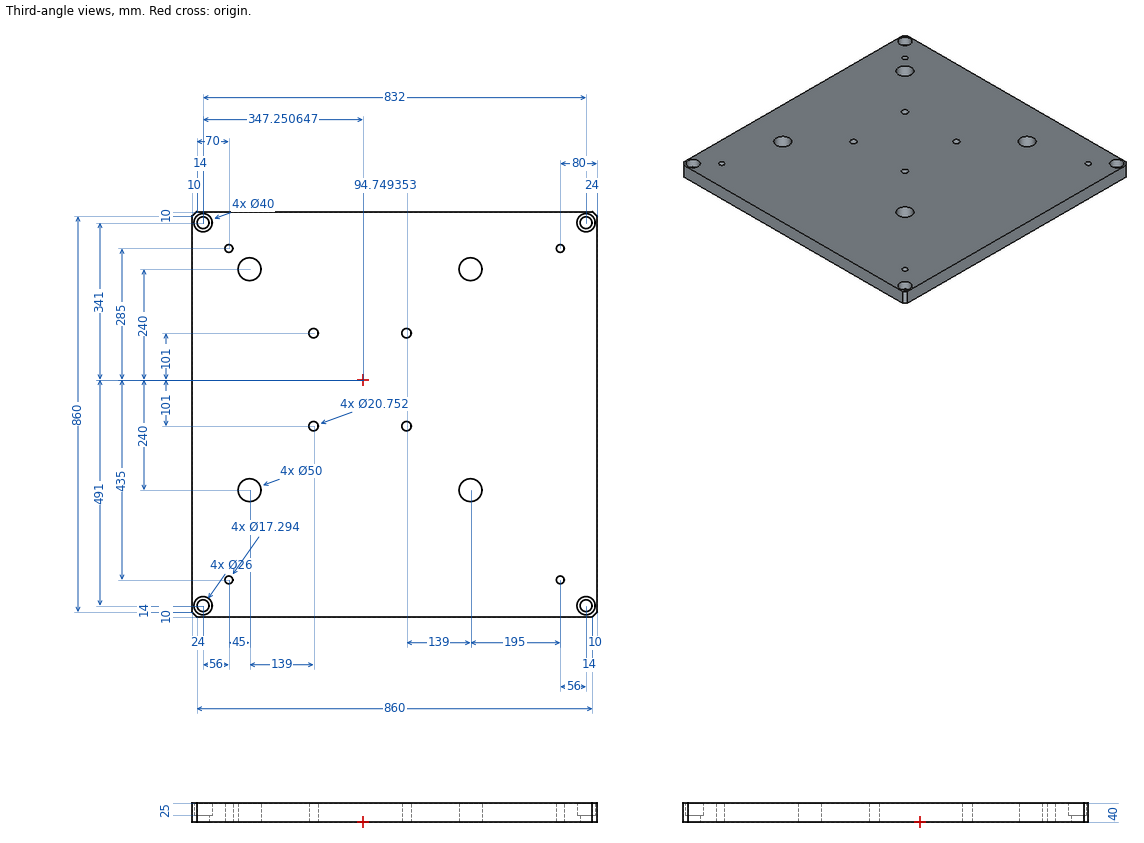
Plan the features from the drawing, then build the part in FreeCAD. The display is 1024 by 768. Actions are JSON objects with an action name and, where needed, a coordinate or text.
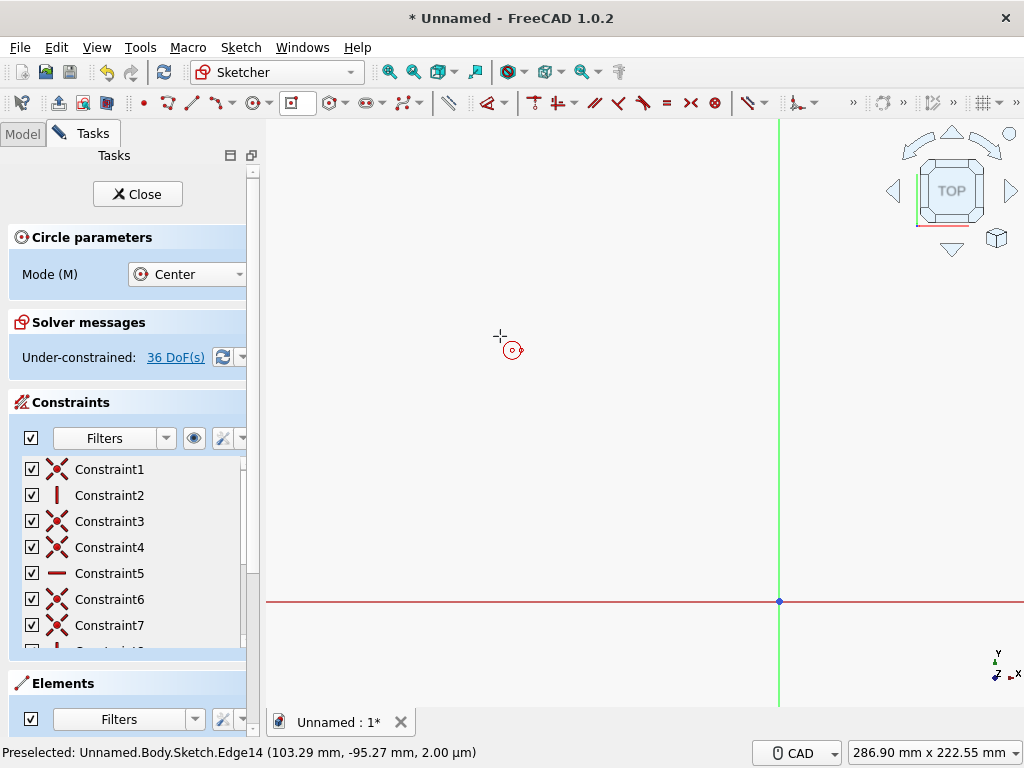
{"action": "scroll", "coordinate": [500, 336], "scroll_direction": "down", "scroll_amount": 9}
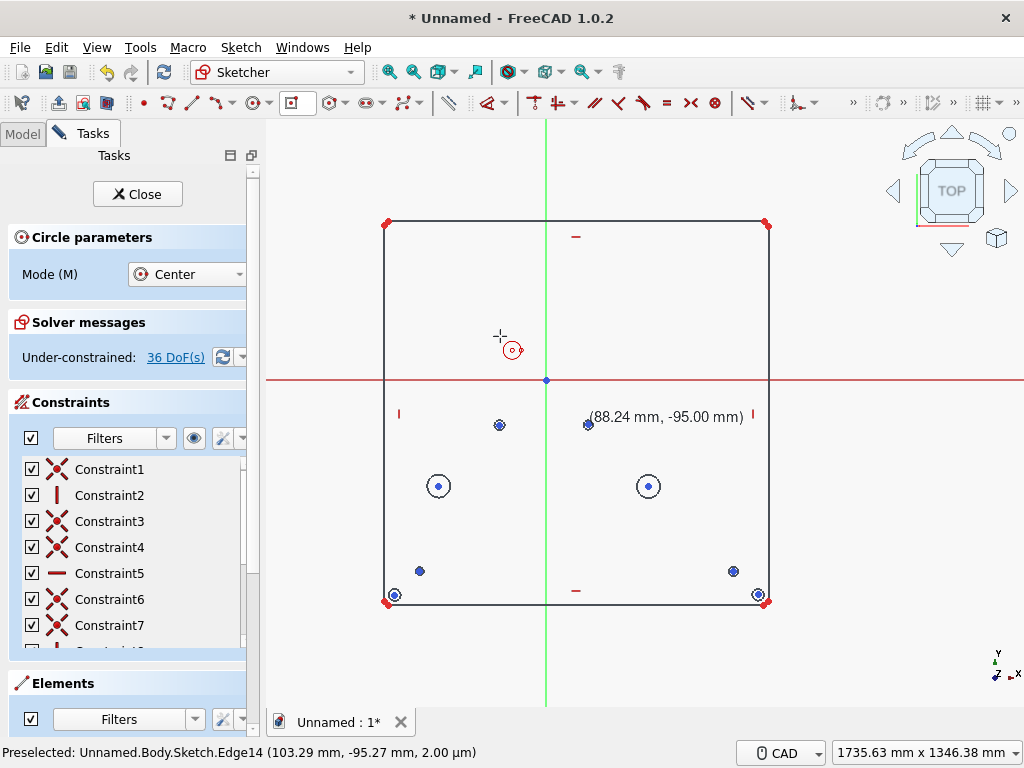
{"action": "left_click", "coordinate": [500, 336]}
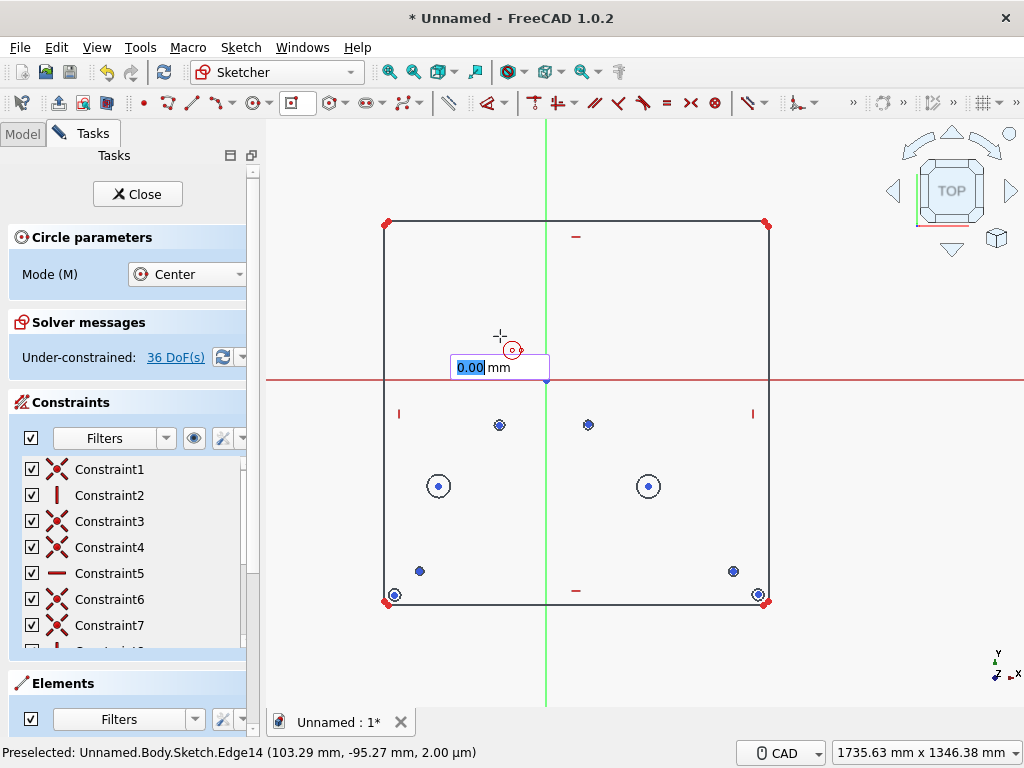
{"action": "scroll", "coordinate": [503, 333], "scroll_direction": "up", "scroll_amount": 7}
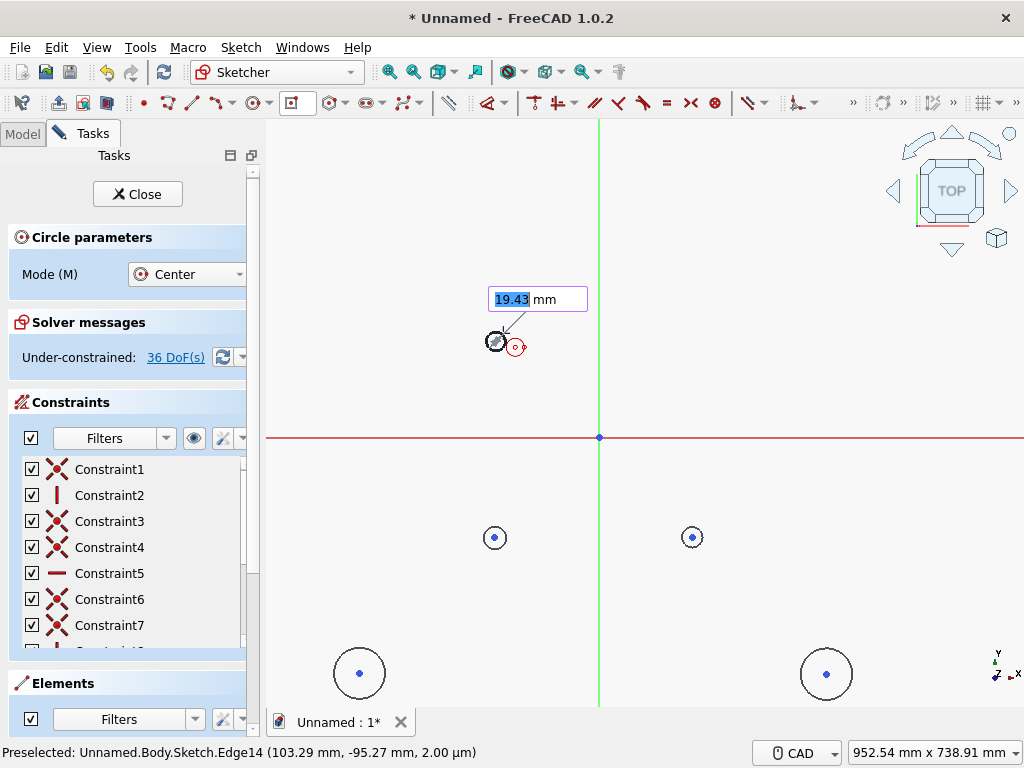
{"action": "left_click", "coordinate": [501, 332]}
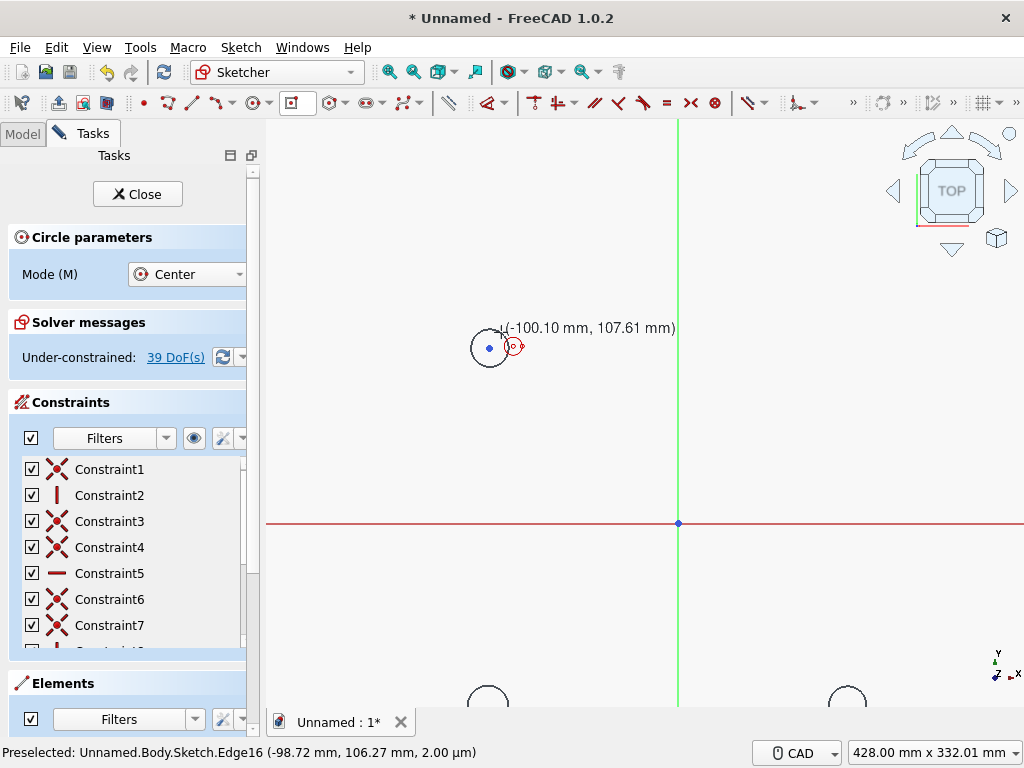
{"action": "scroll", "coordinate": [503, 333], "scroll_direction": "down", "scroll_amount": 7}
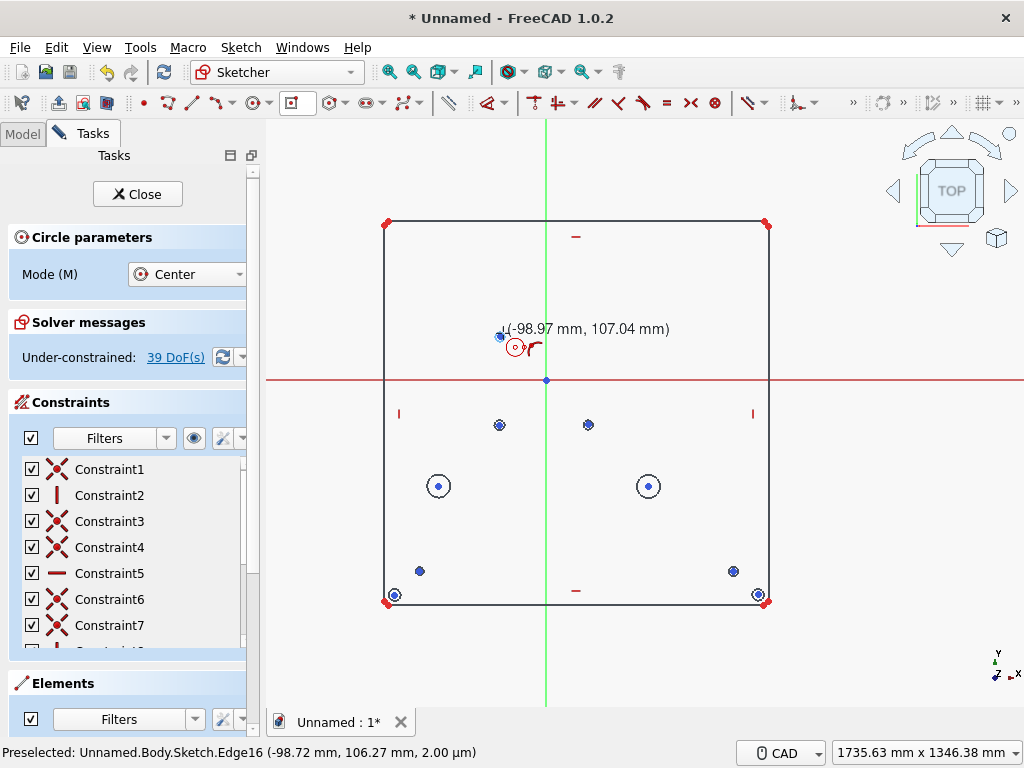
{"action": "scroll", "coordinate": [439, 275], "scroll_direction": "up", "scroll_amount": 4}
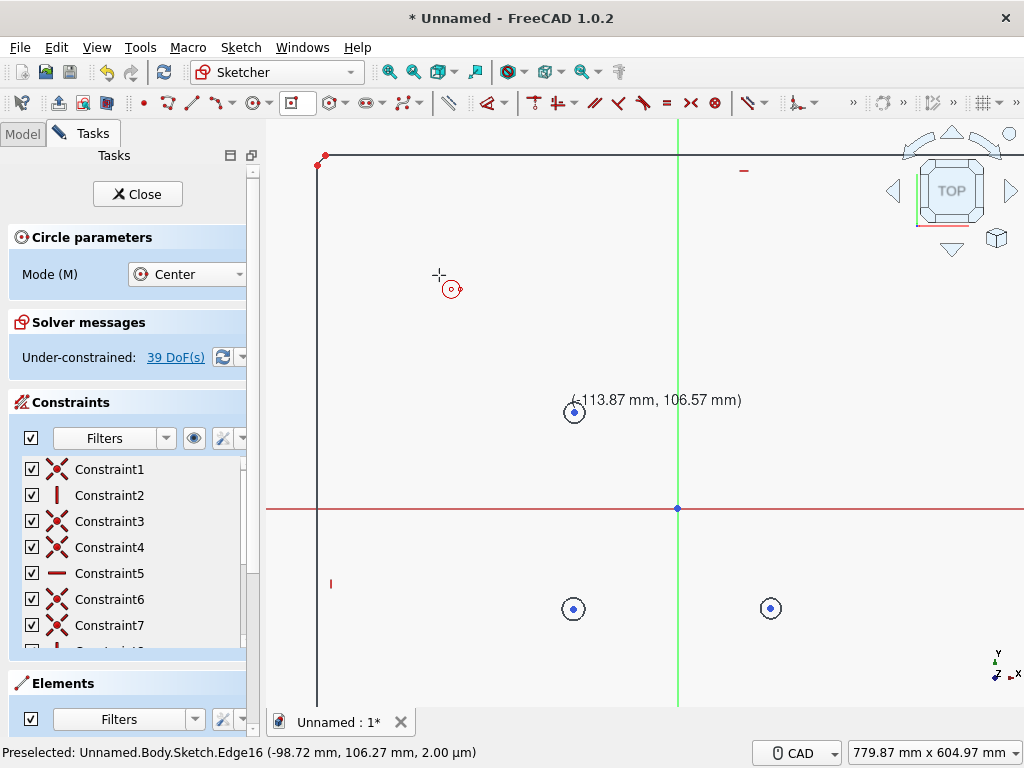
{"action": "left_click", "coordinate": [439, 276]}
{"action": "left_click", "coordinate": [456, 259]}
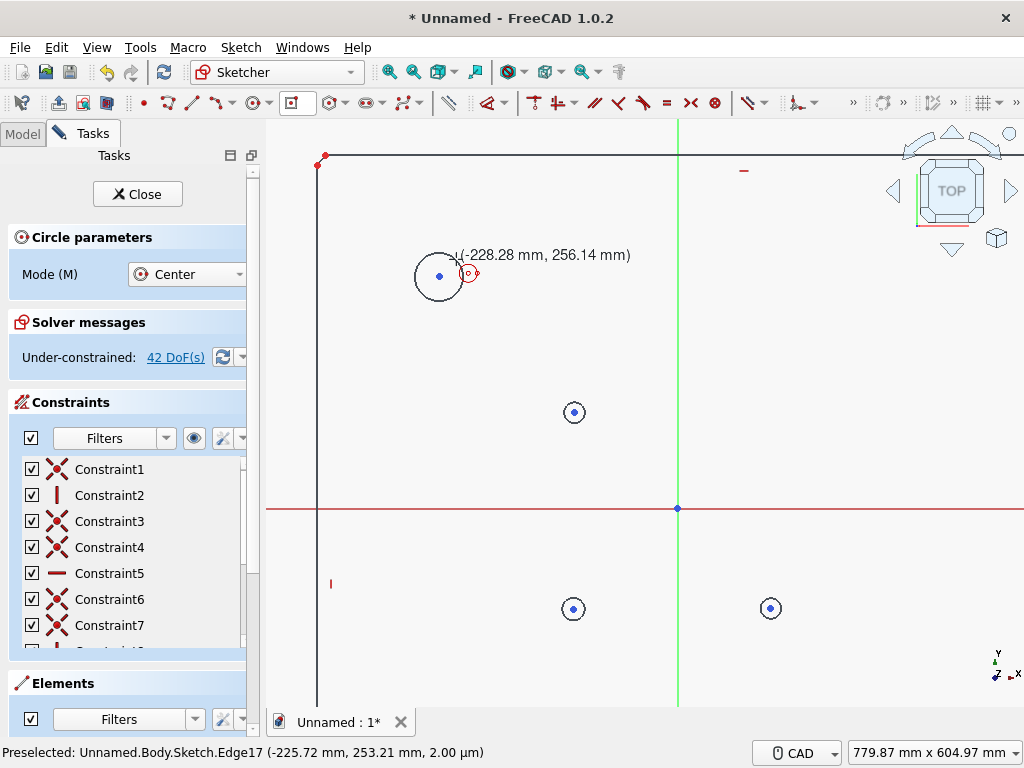
{"action": "scroll", "coordinate": [395, 232], "scroll_direction": "up", "scroll_amount": 5}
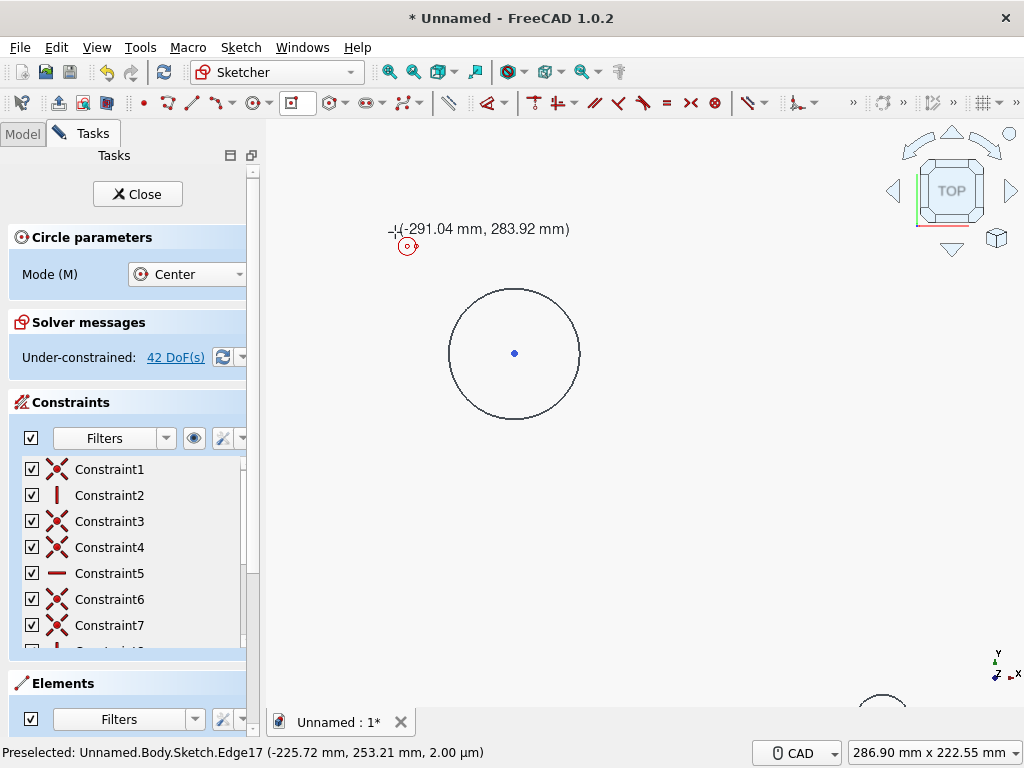
{"action": "scroll", "coordinate": [424, 261], "scroll_direction": "down", "scroll_amount": 9}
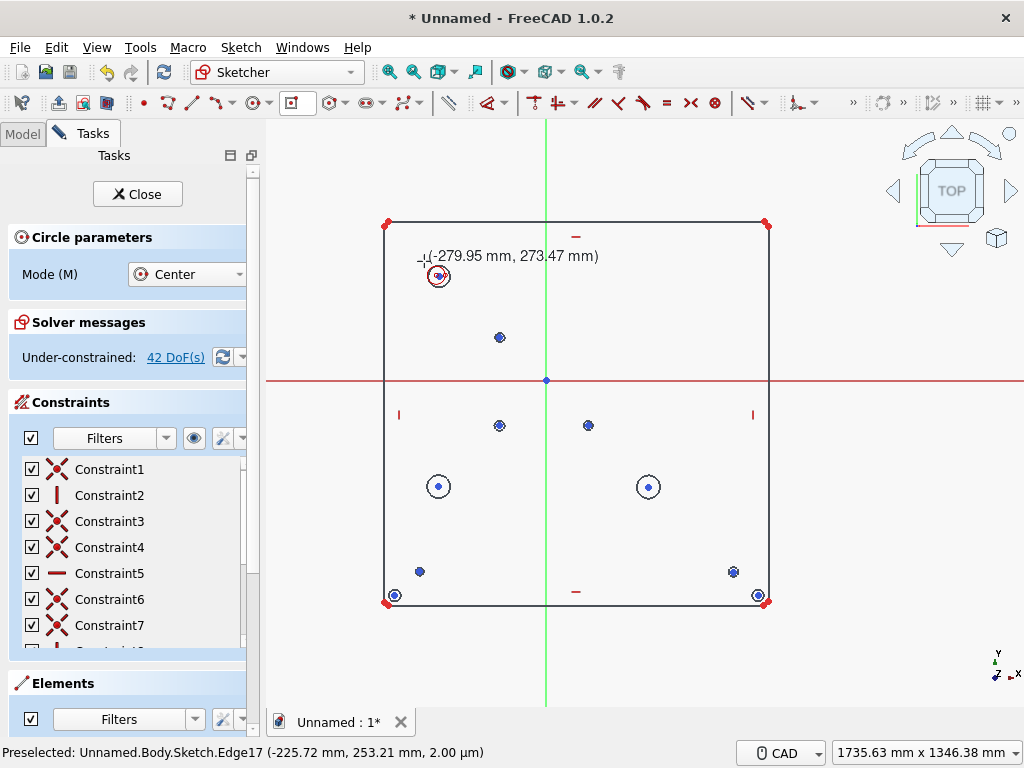
{"action": "left_click", "coordinate": [419, 256]}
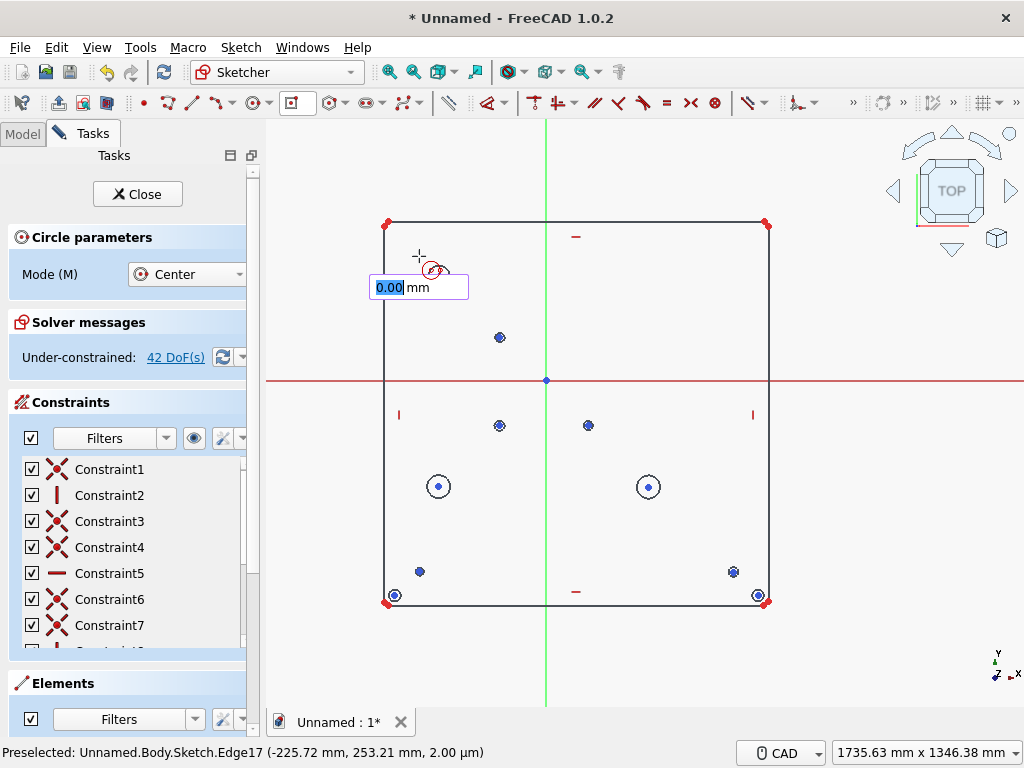
{"action": "scroll", "coordinate": [422, 254], "scroll_direction": "up", "scroll_amount": 8}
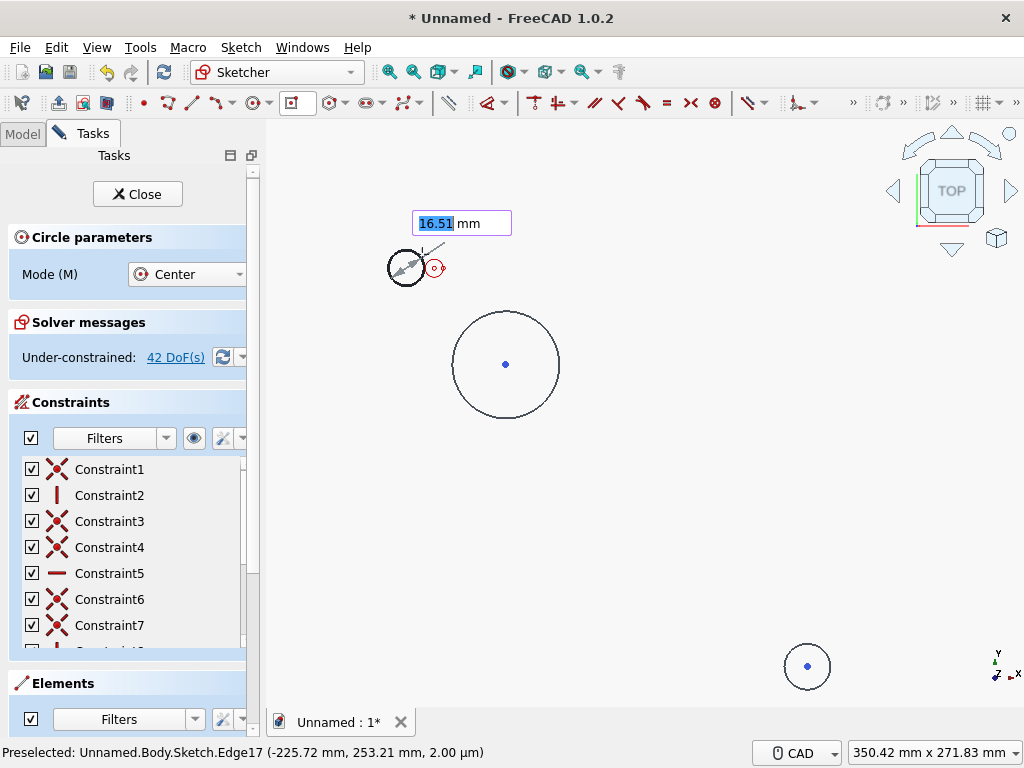
{"action": "left_click", "coordinate": [421, 251]}